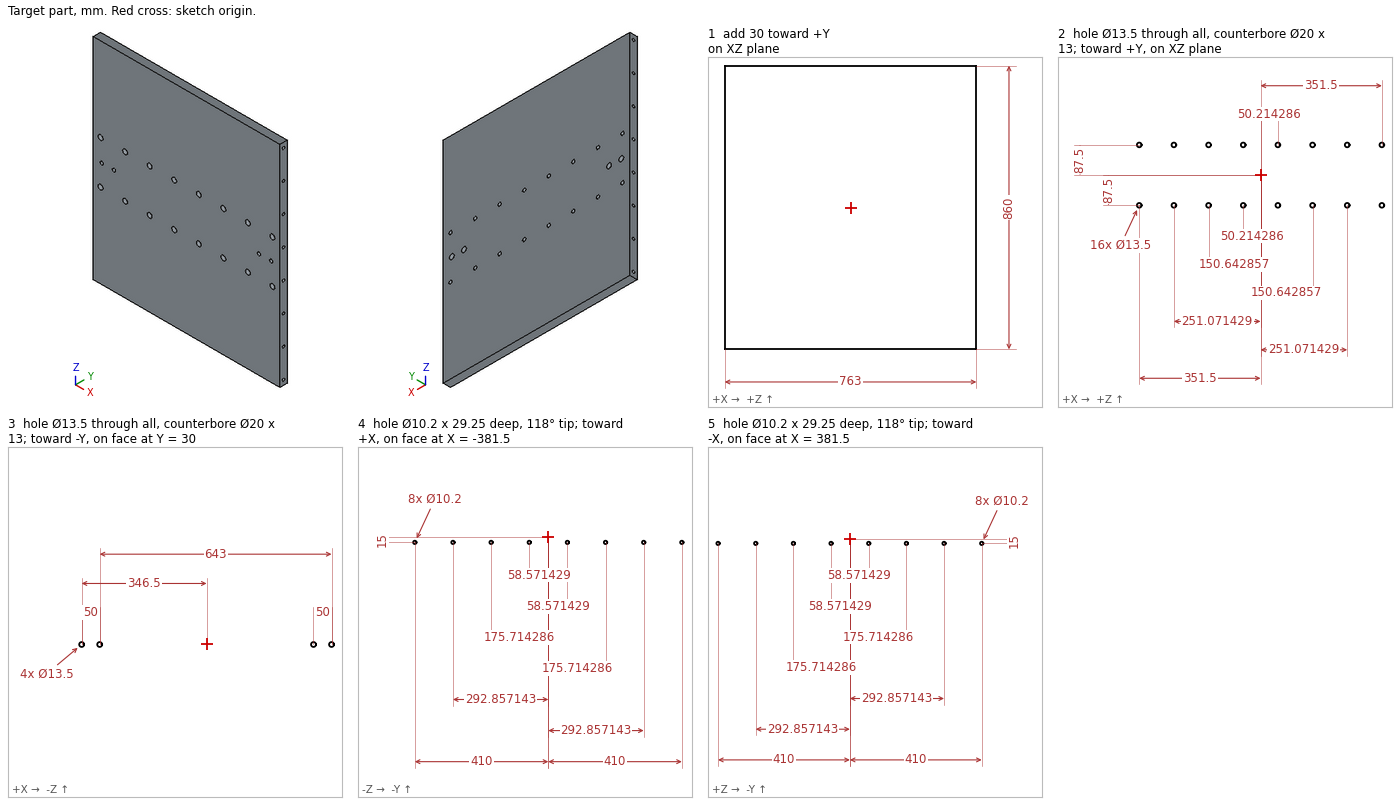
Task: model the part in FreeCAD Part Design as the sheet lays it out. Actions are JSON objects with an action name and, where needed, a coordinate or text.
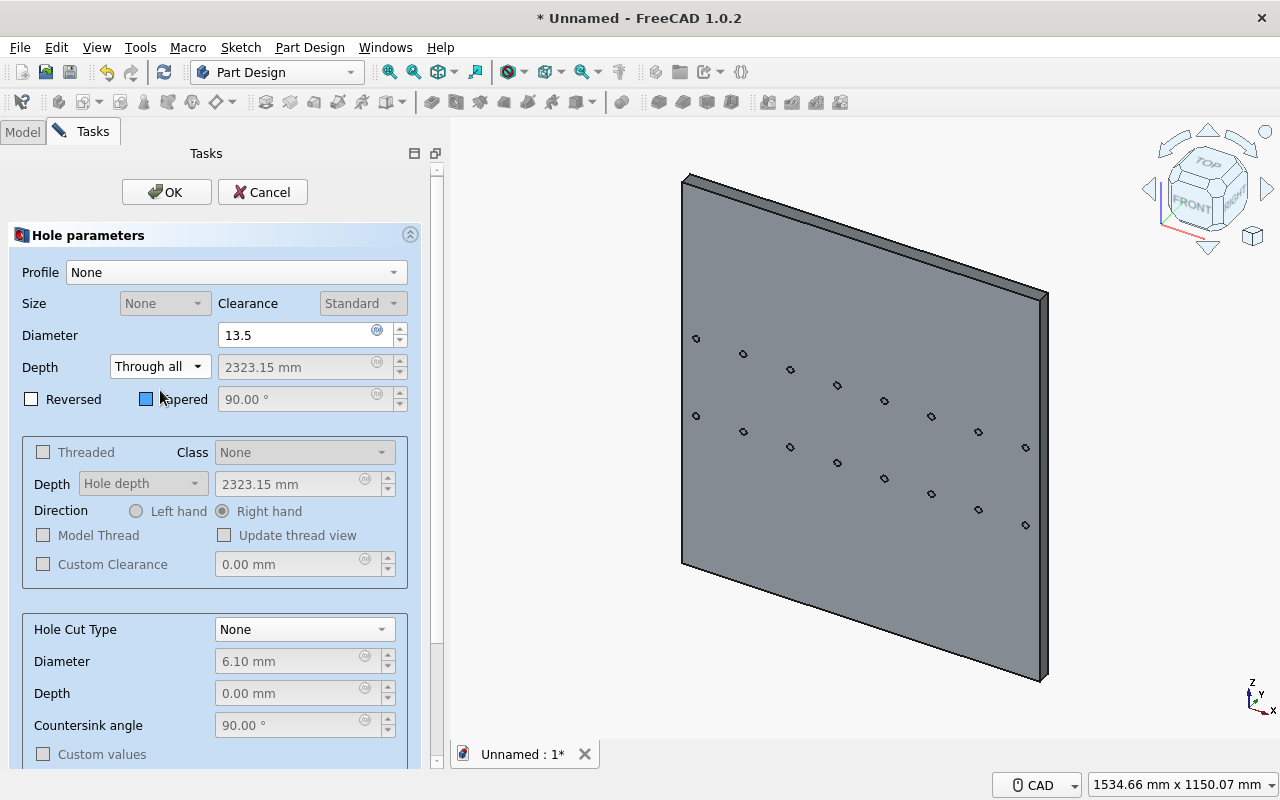
{"action": "left_click", "coordinate": [306, 630]}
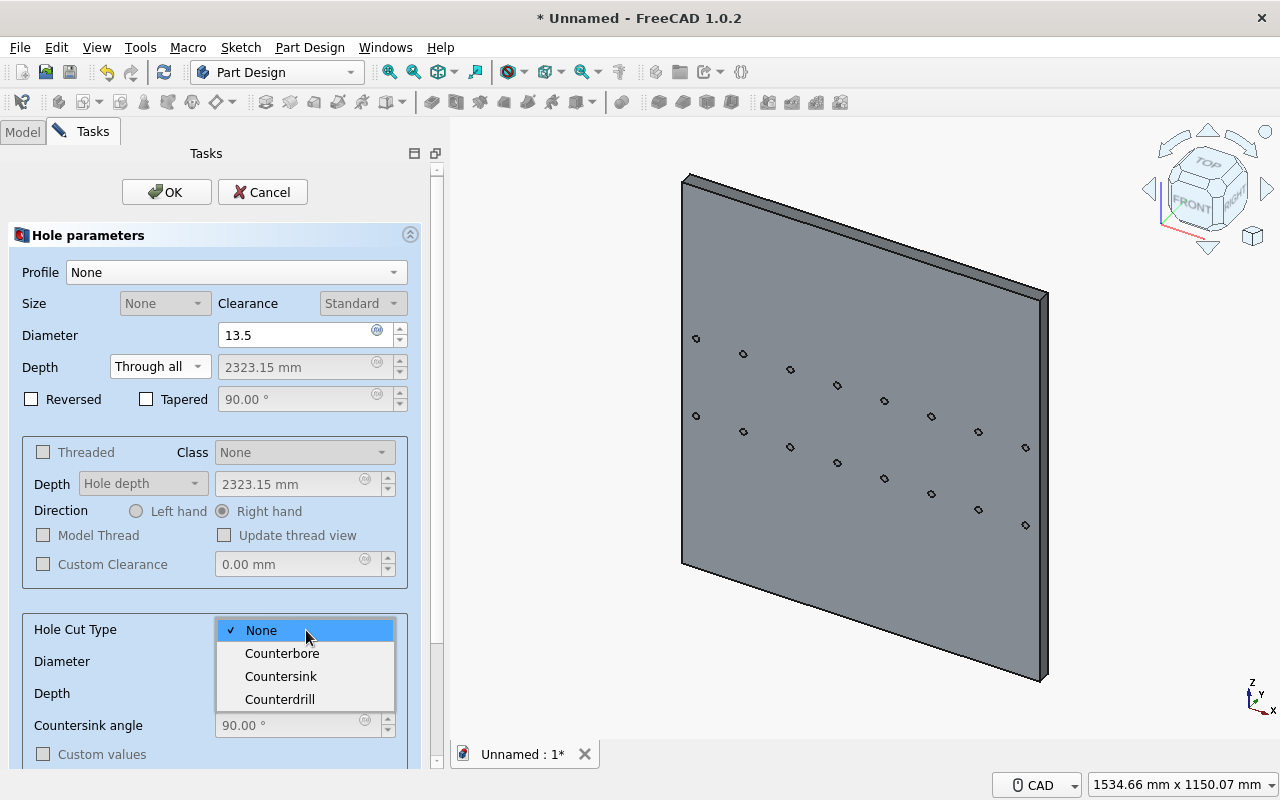
{"action": "left_click", "coordinate": [304, 654]}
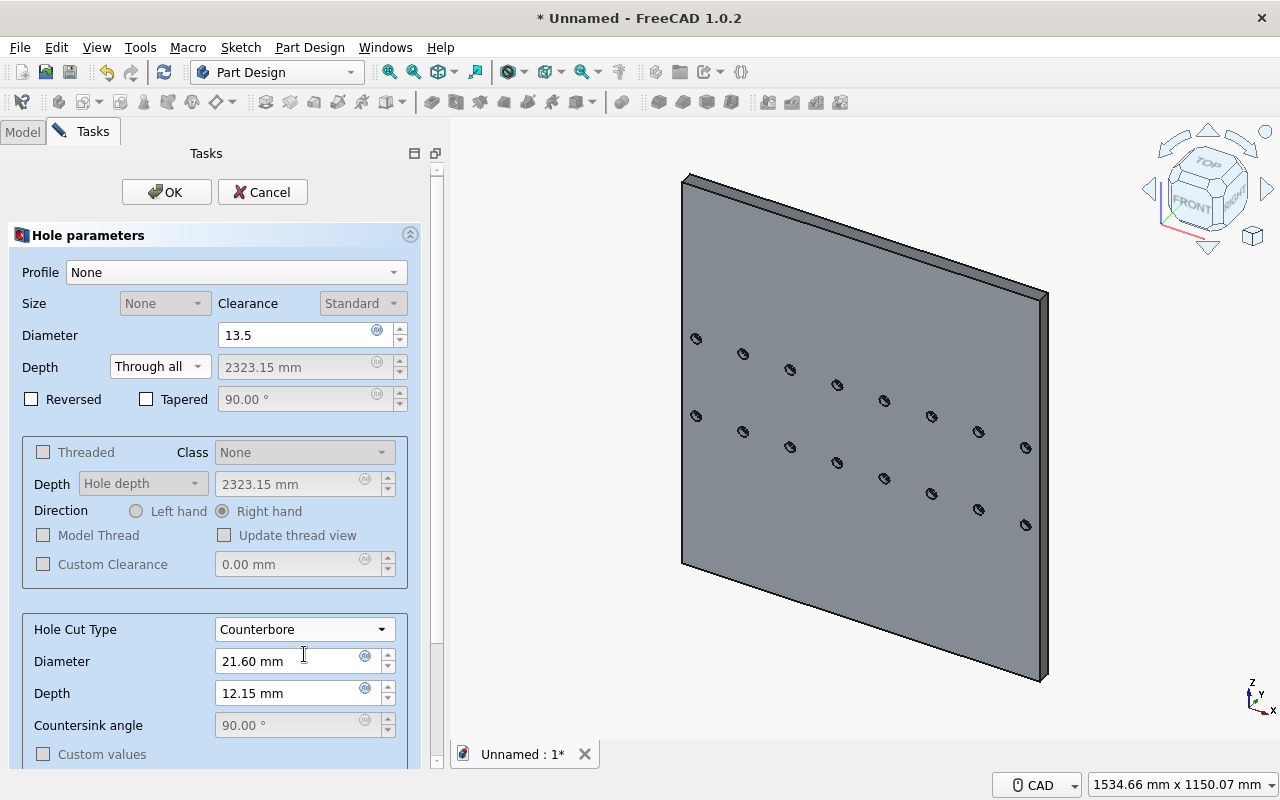
{"action": "triple_click", "coordinate": [298, 661]}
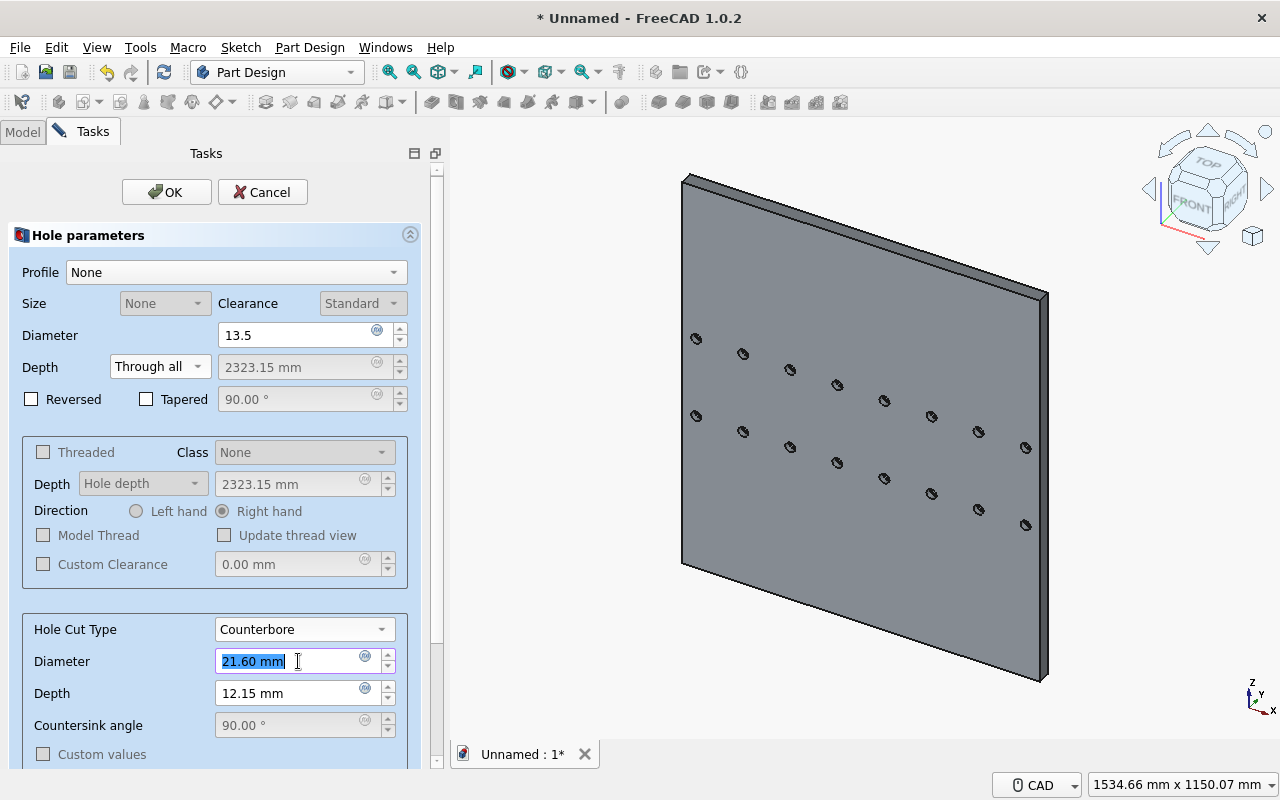
{"action": "type", "text": "20"}
{"action": "key", "text": "Tab"}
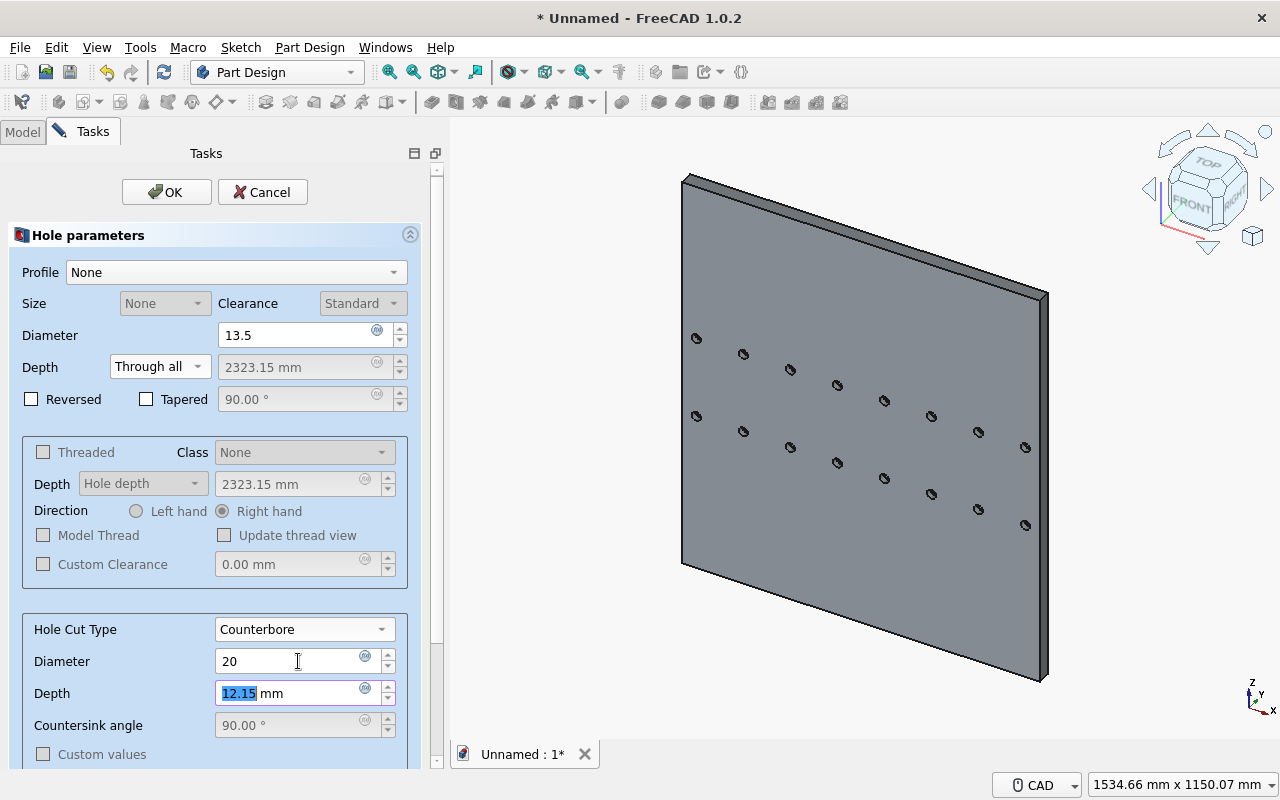
{"action": "type", "text": "13"}
{"action": "key", "text": "Tab"}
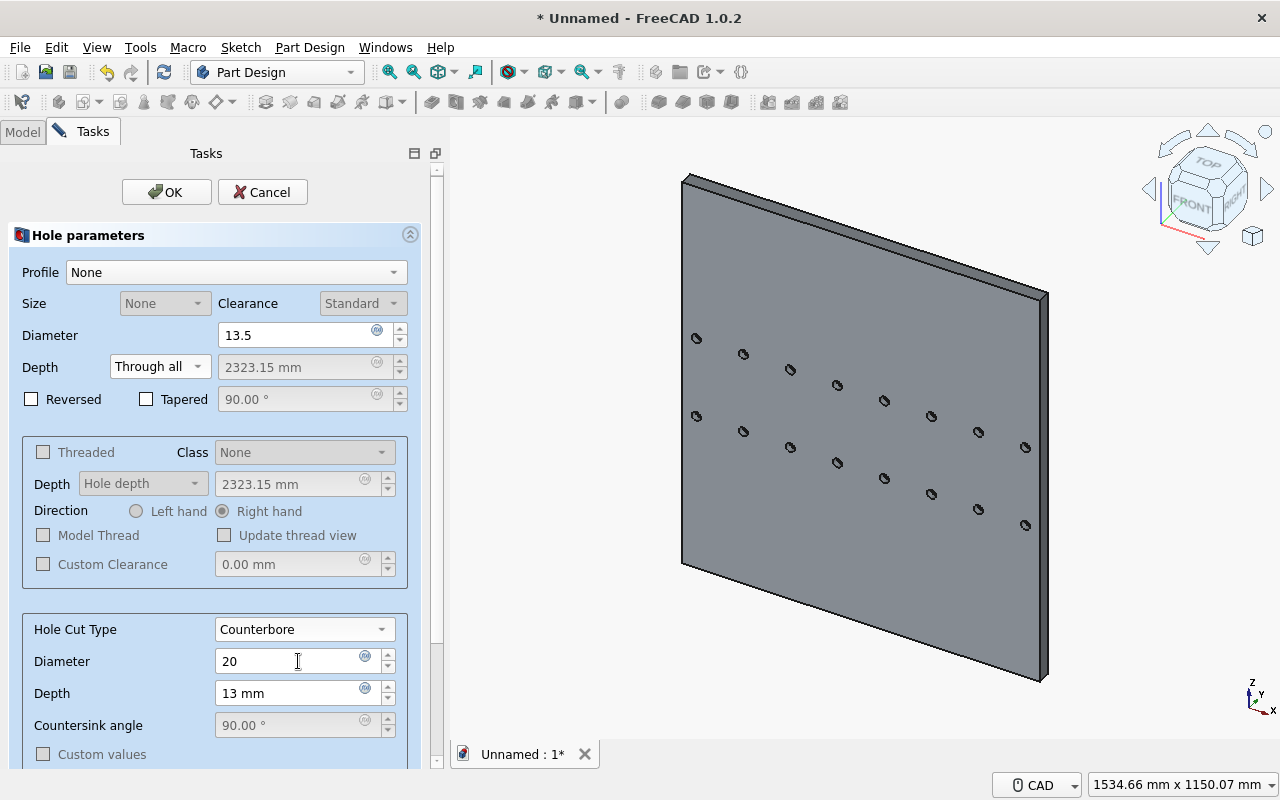
{"action": "left_click", "coordinate": [167, 192]}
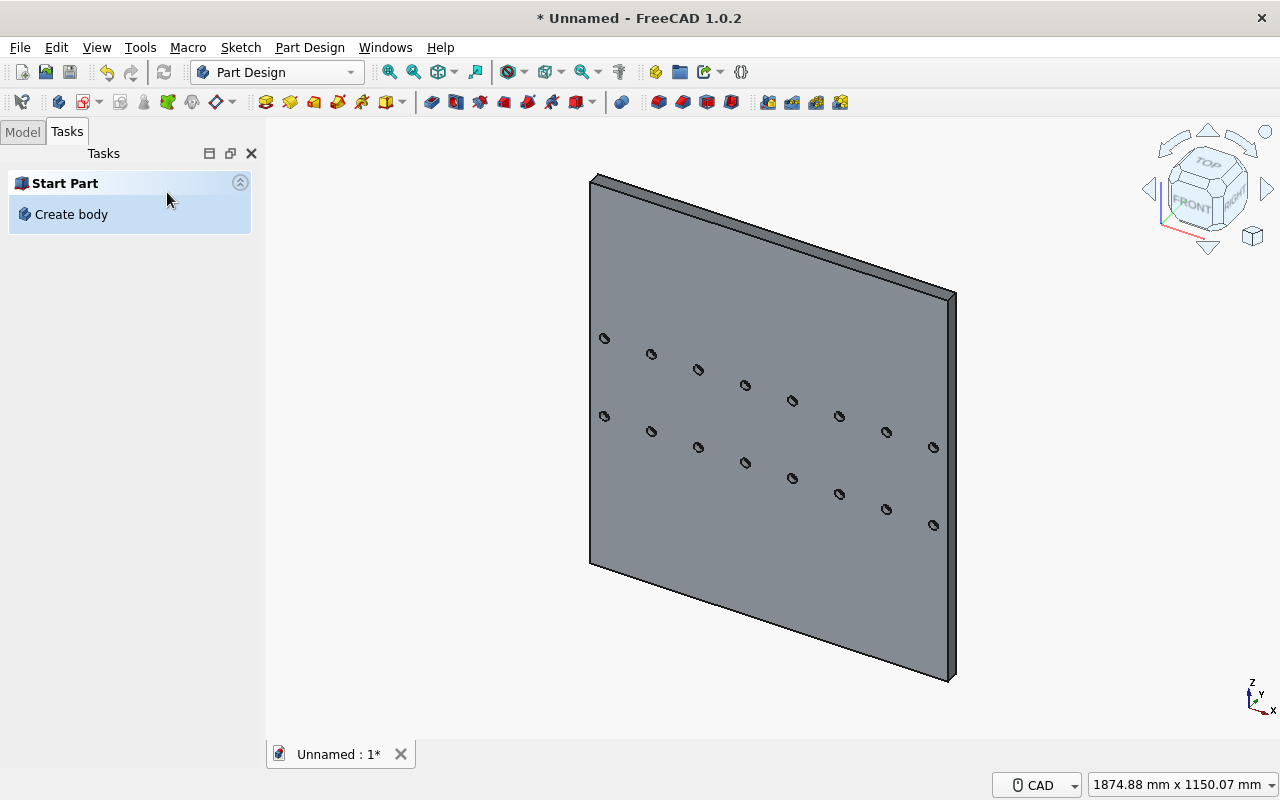
{"action": "key", "text": "4"}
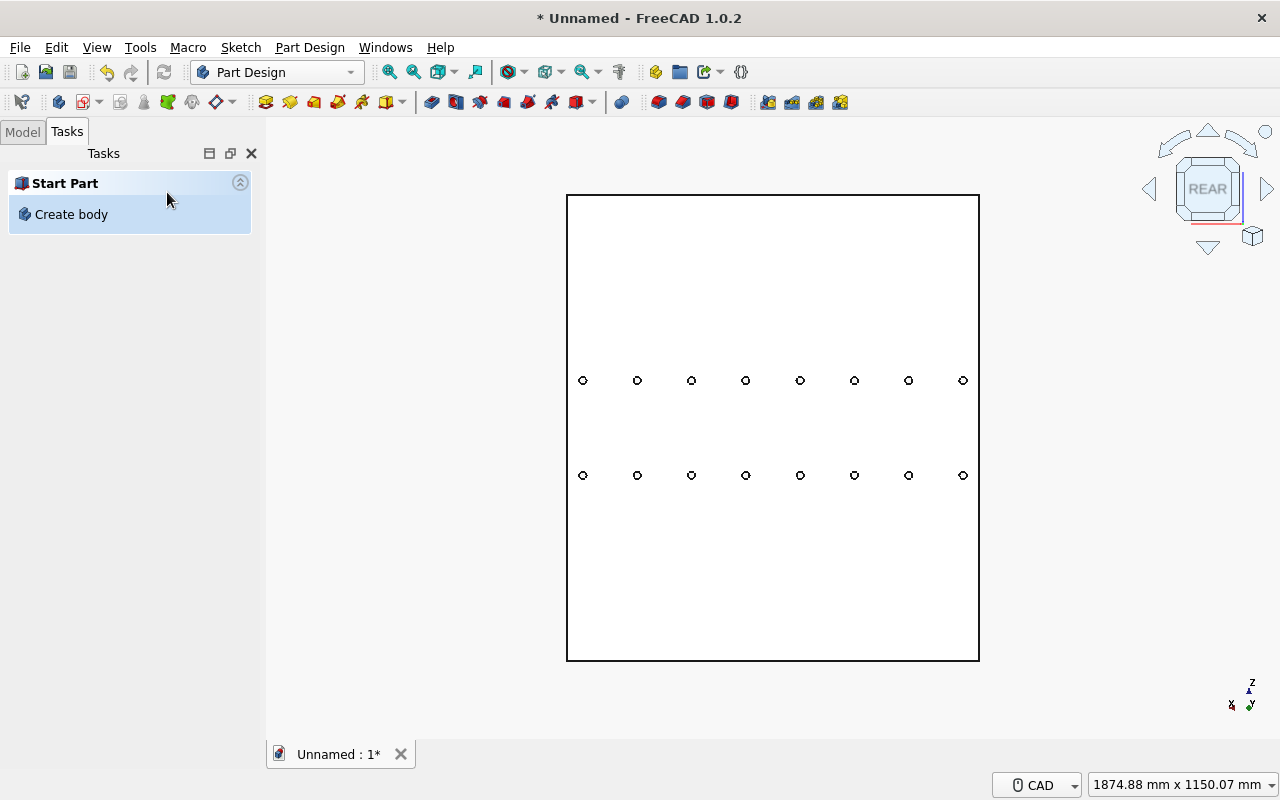
{"action": "left_click", "coordinate": [773, 294]}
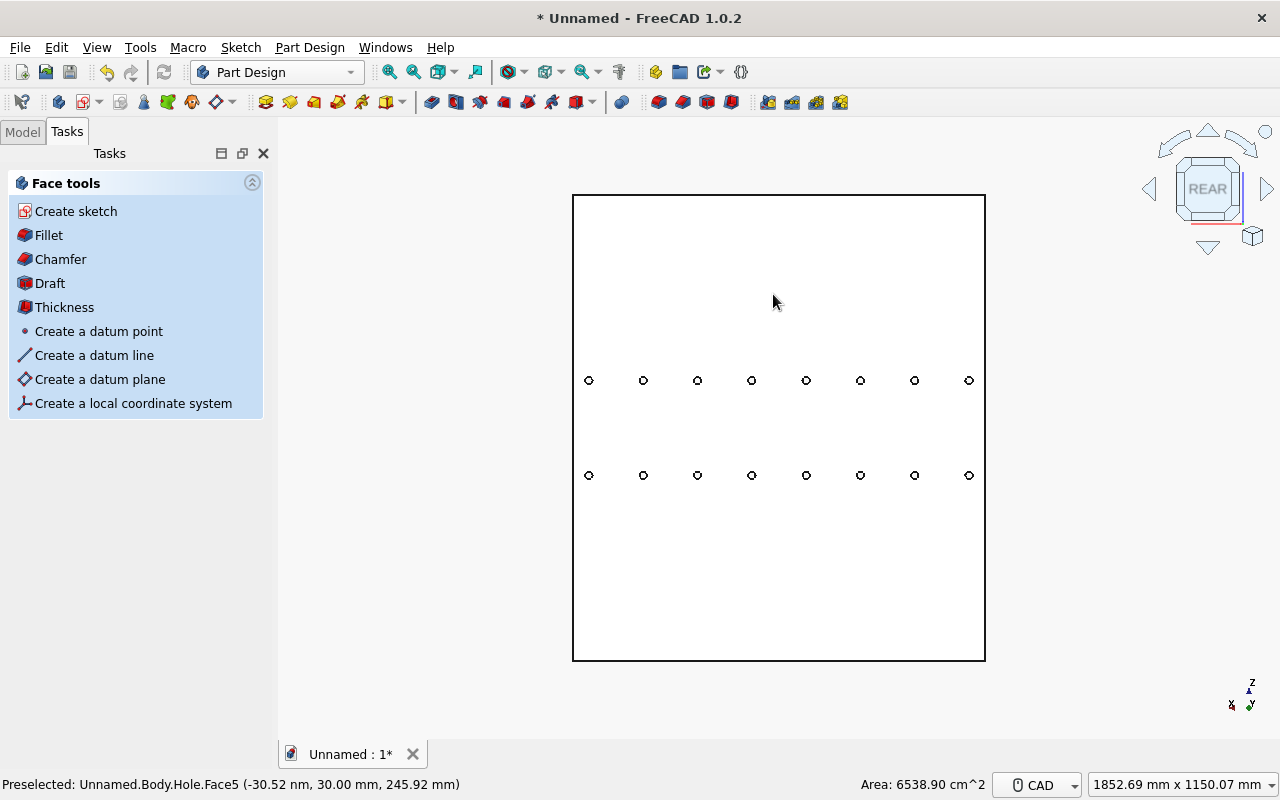
{"action": "left_click", "coordinate": [84, 102]}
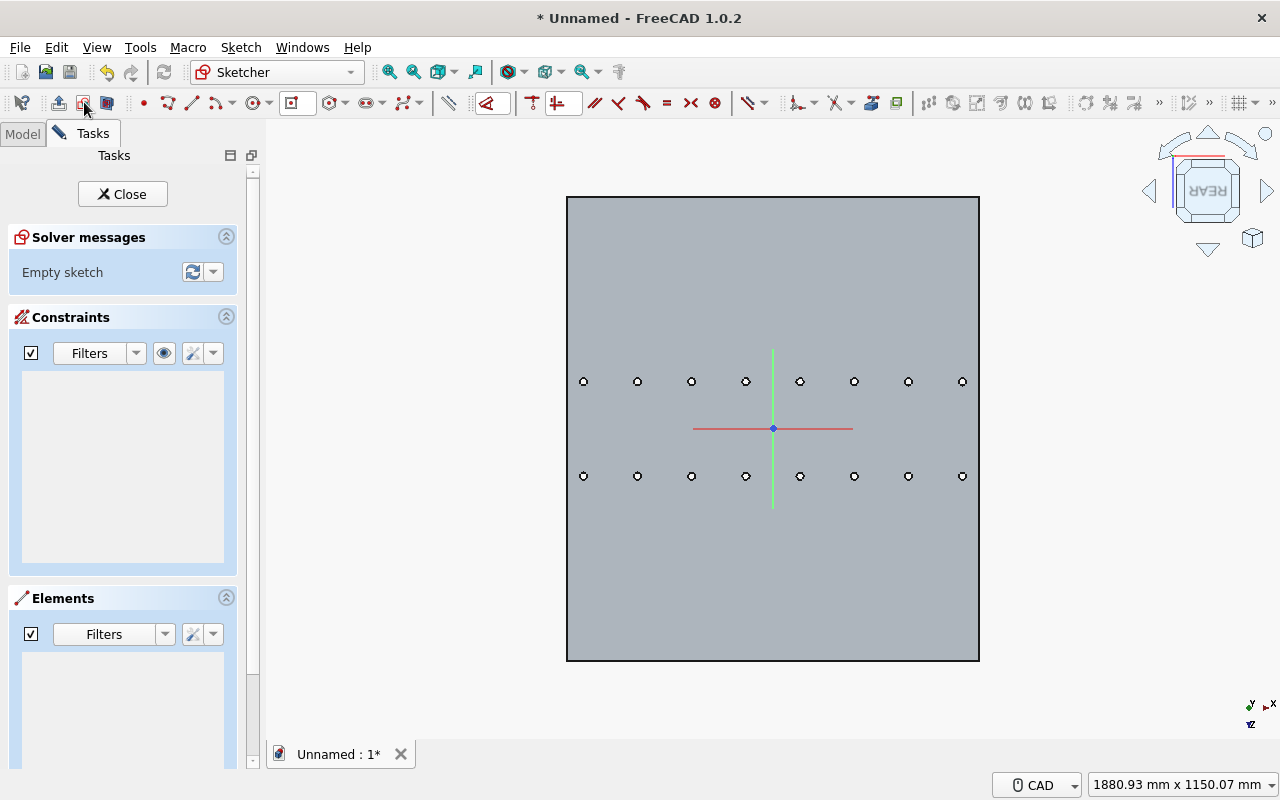
{"action": "scroll", "coordinate": [912, 429], "scroll_direction": "up", "scroll_amount": 2}